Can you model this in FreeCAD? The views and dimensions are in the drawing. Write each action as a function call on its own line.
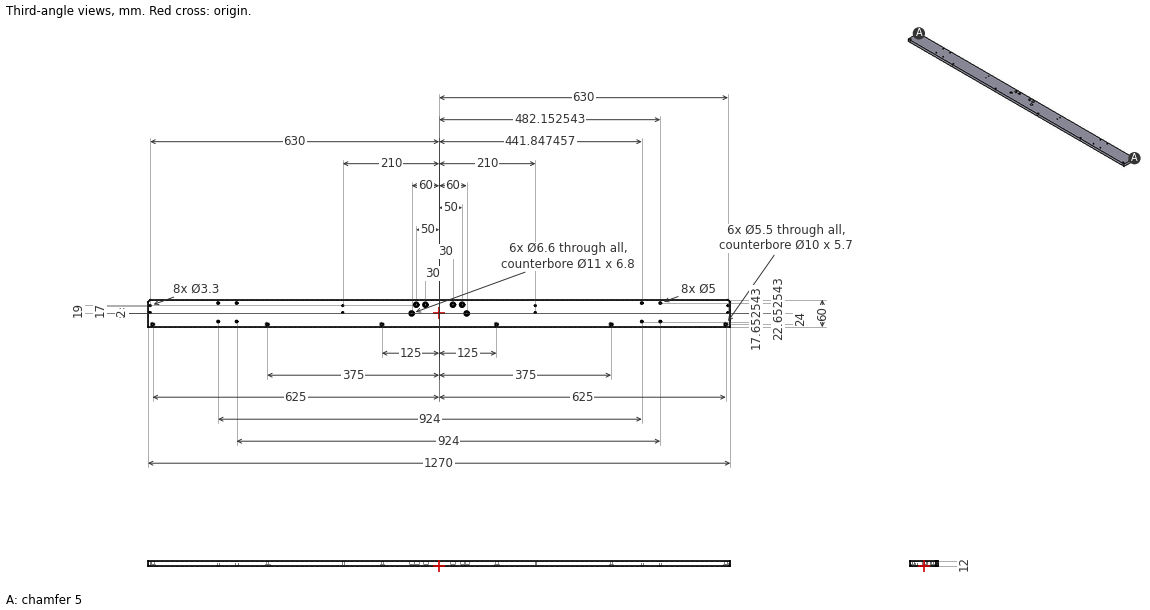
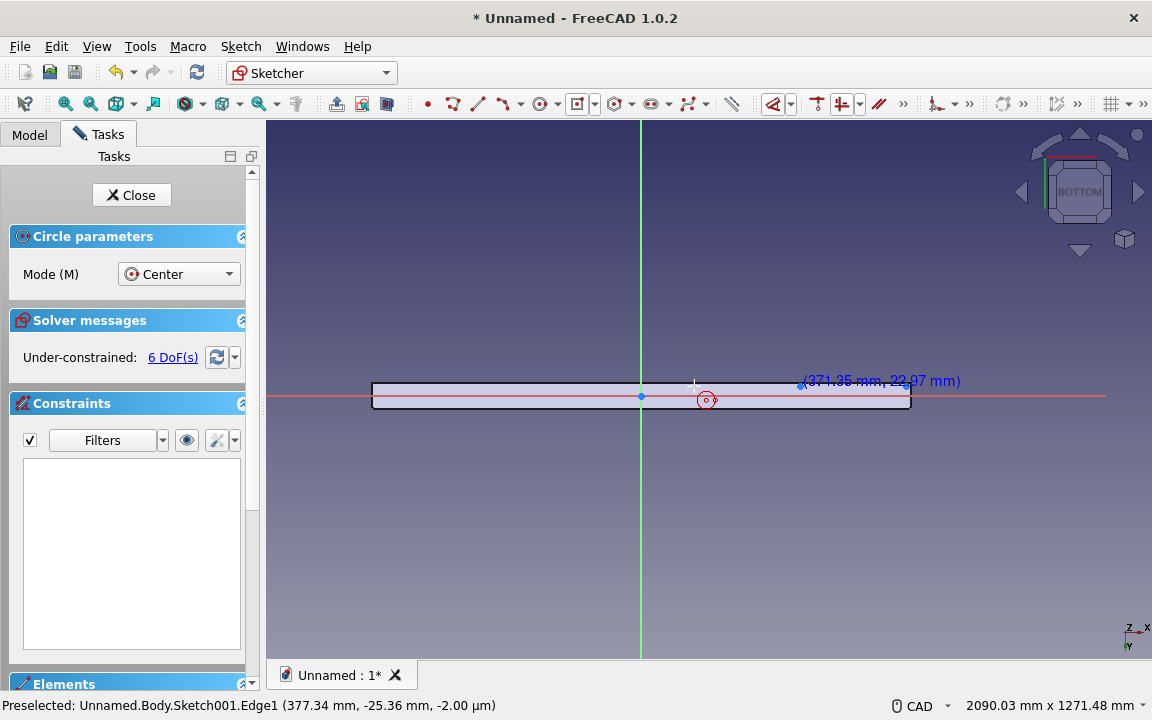
scroll(694, 386, up, 3)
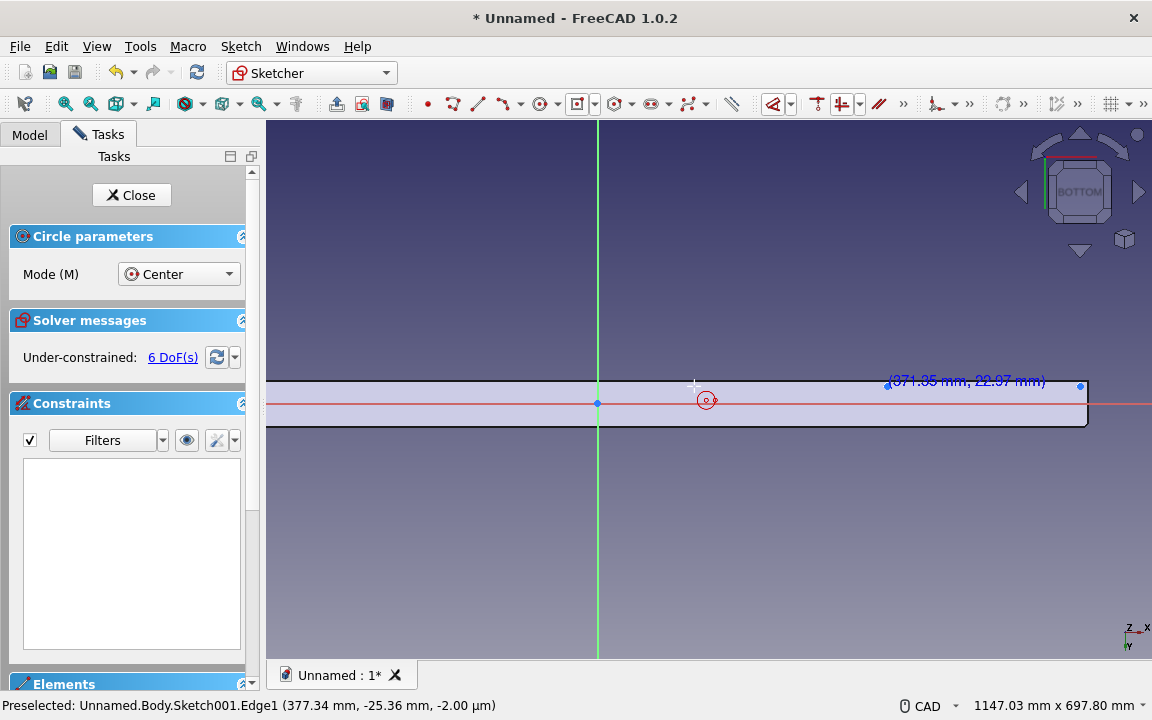
click(694, 385)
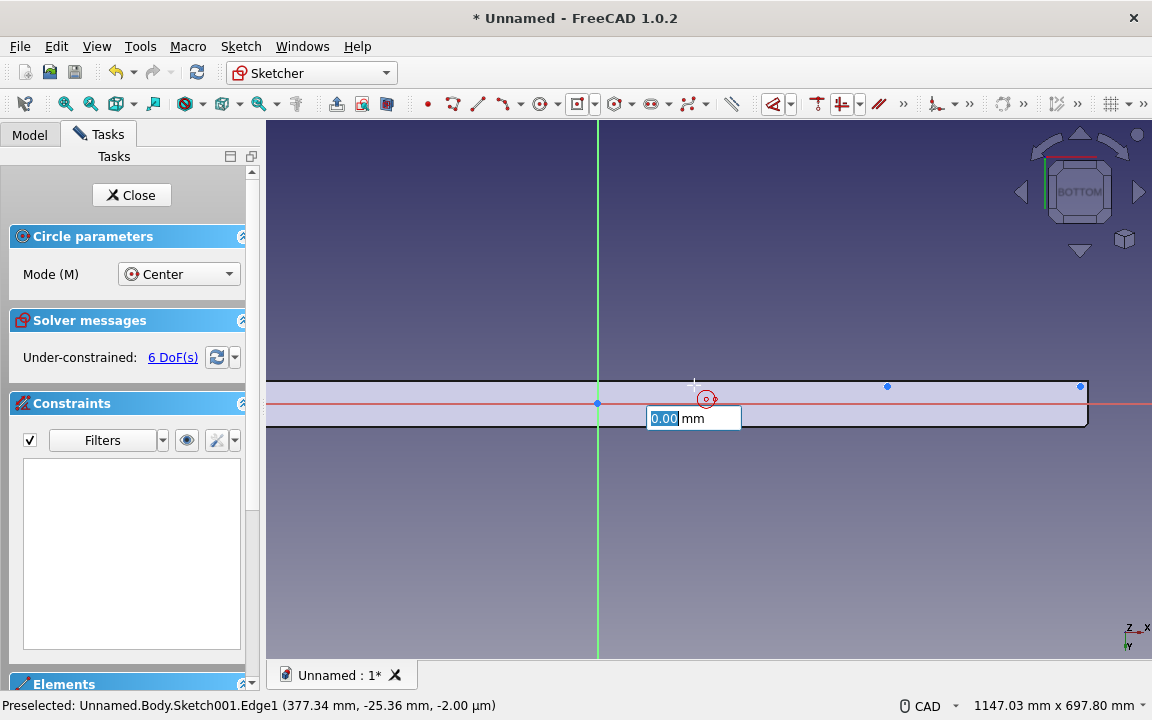
scroll(696, 384, up, 11)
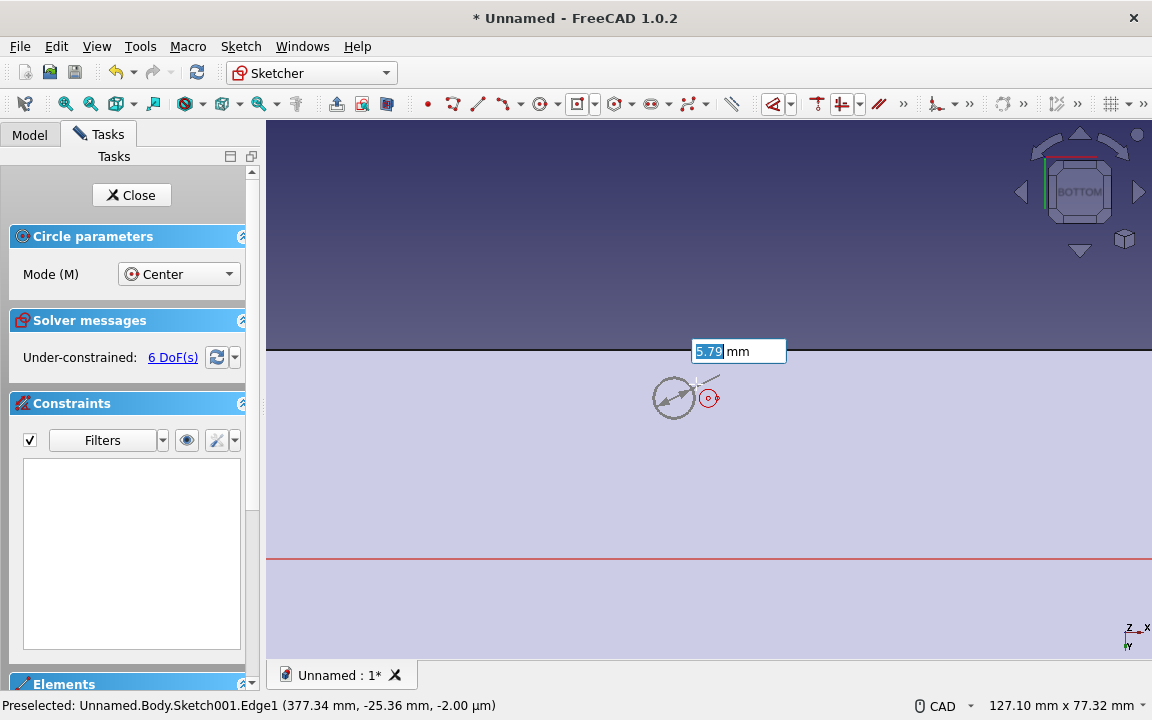
click(689, 378)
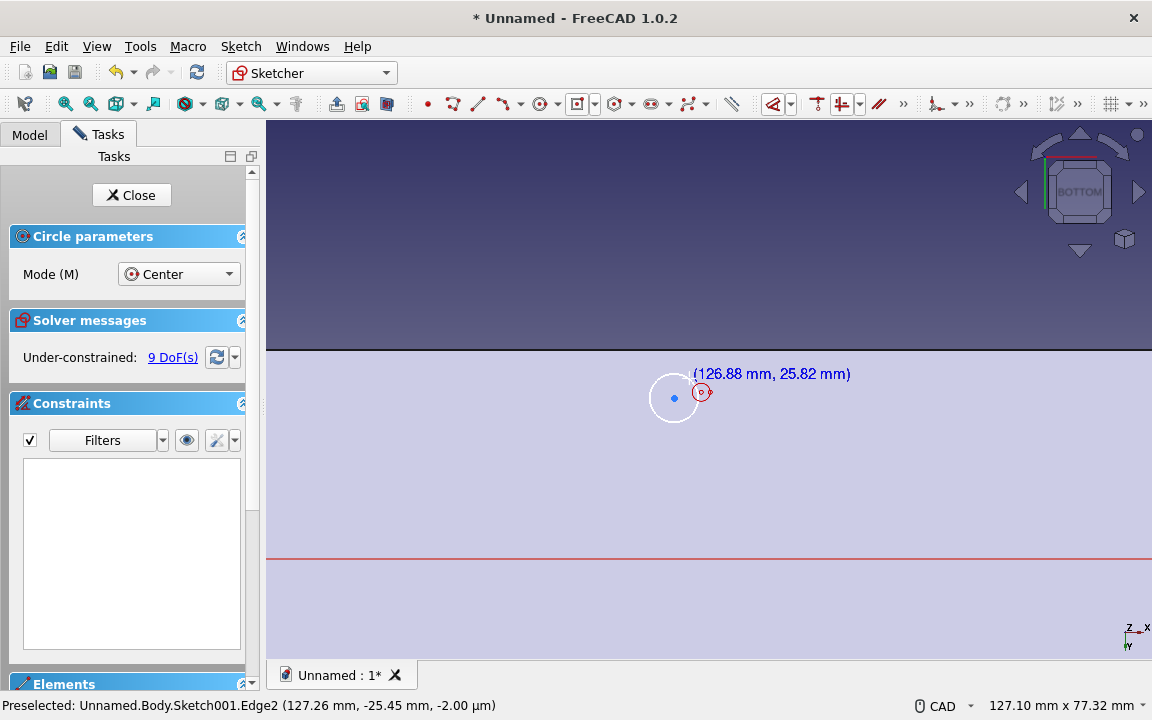
scroll(695, 385, down, 14)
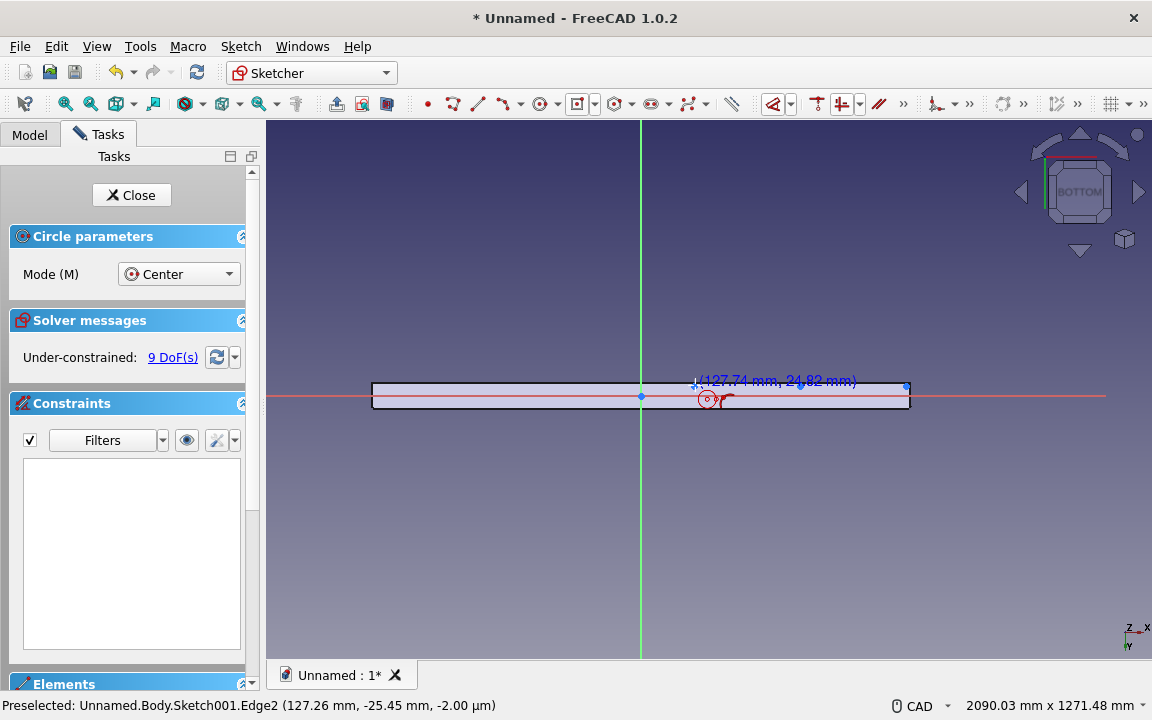
scroll(588, 386, up, 15)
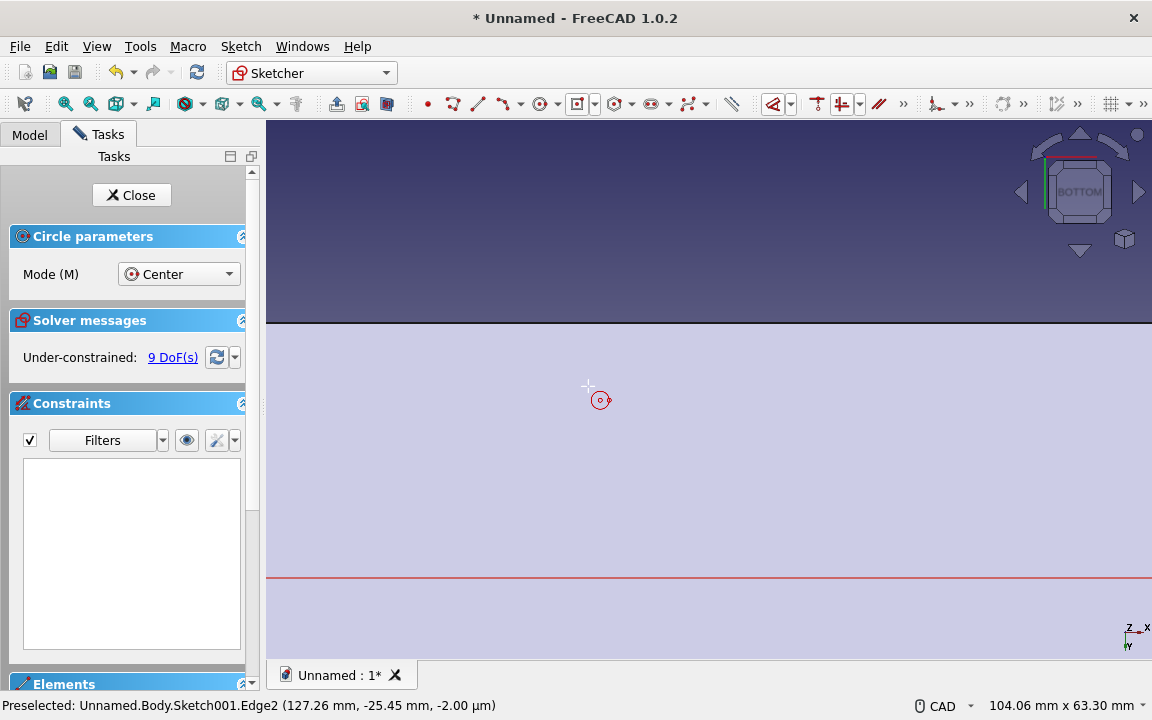
scroll(588, 386, down, 15)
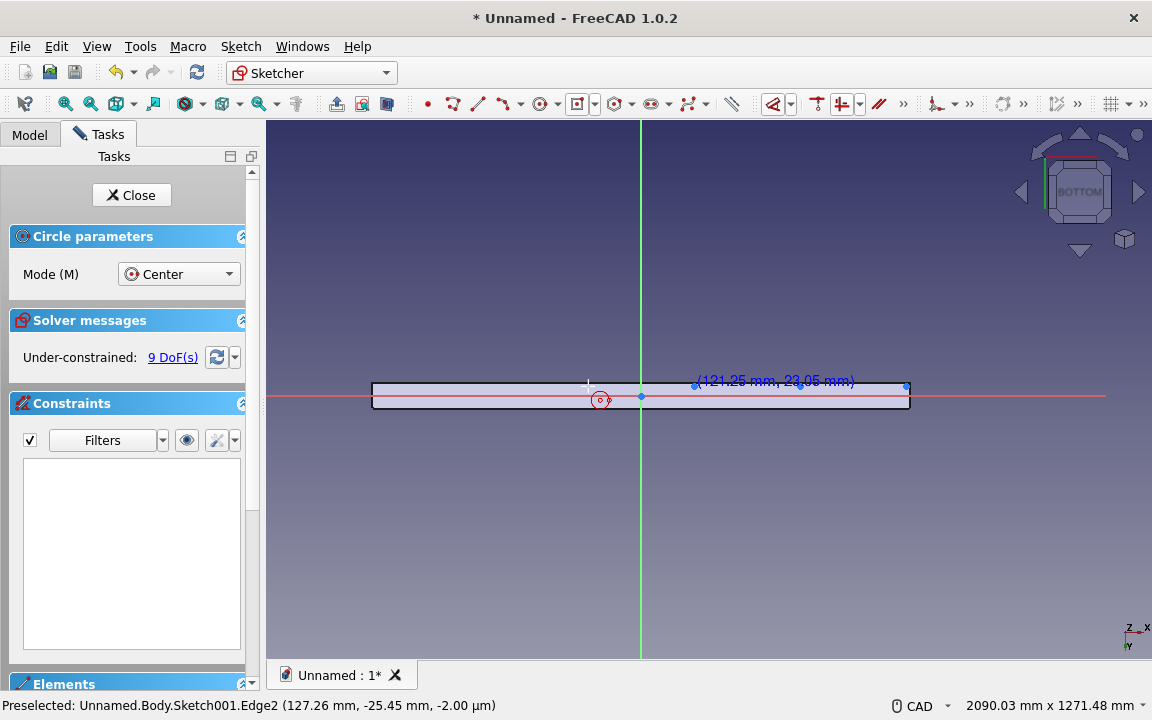
scroll(588, 386, up, 3)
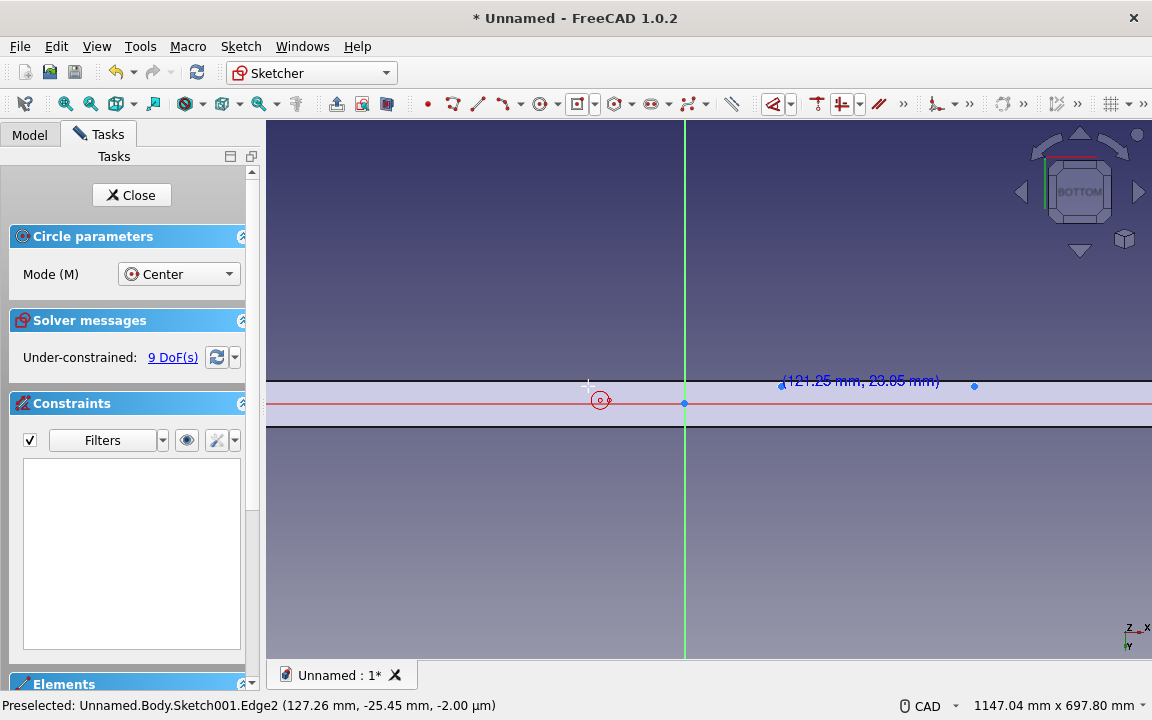
click(588, 385)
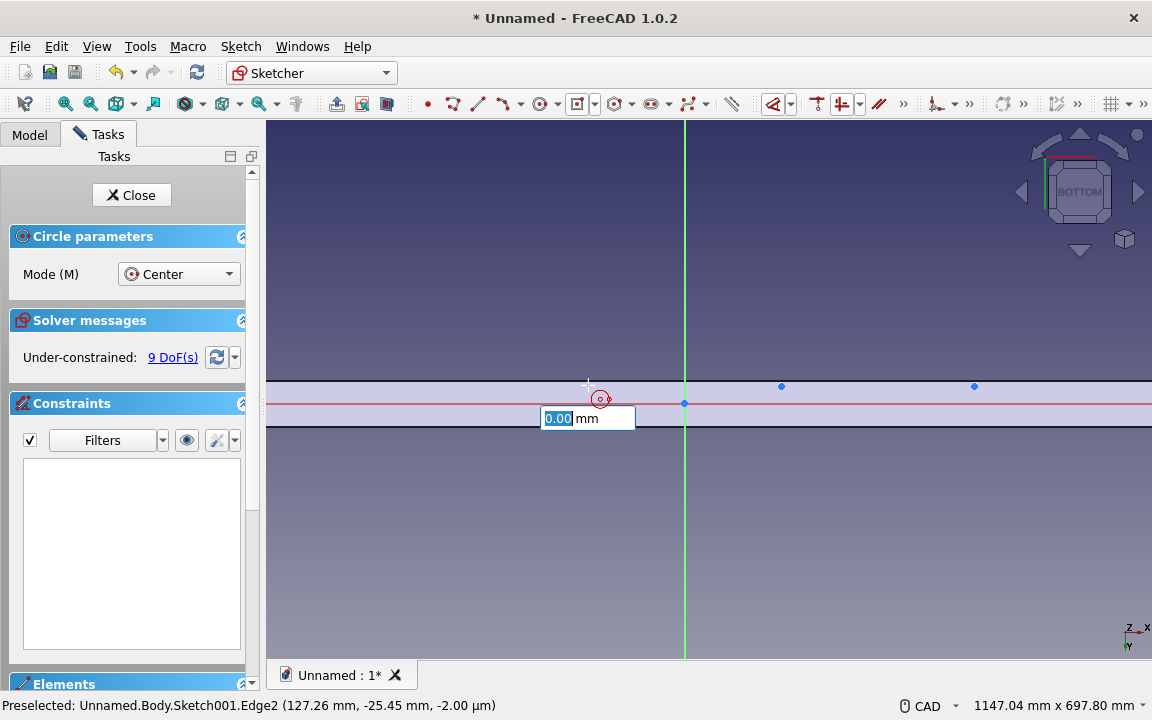
scroll(590, 384, up, 11)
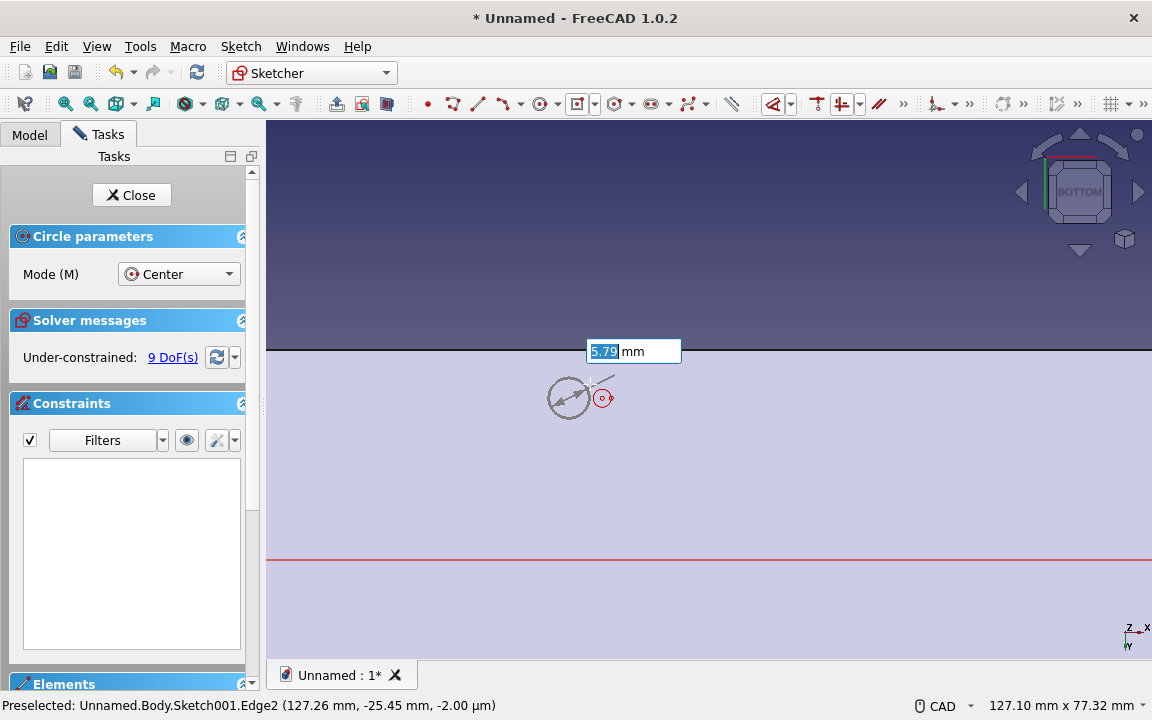
click(585, 379)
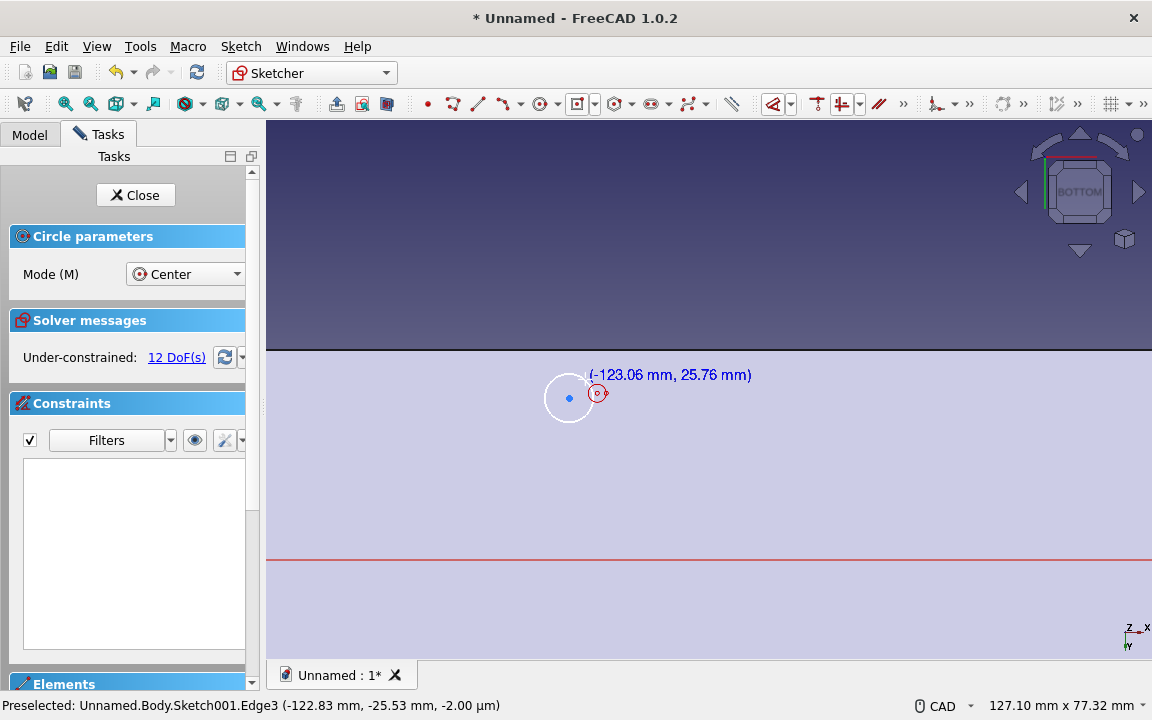
scroll(589, 385, down, 14)